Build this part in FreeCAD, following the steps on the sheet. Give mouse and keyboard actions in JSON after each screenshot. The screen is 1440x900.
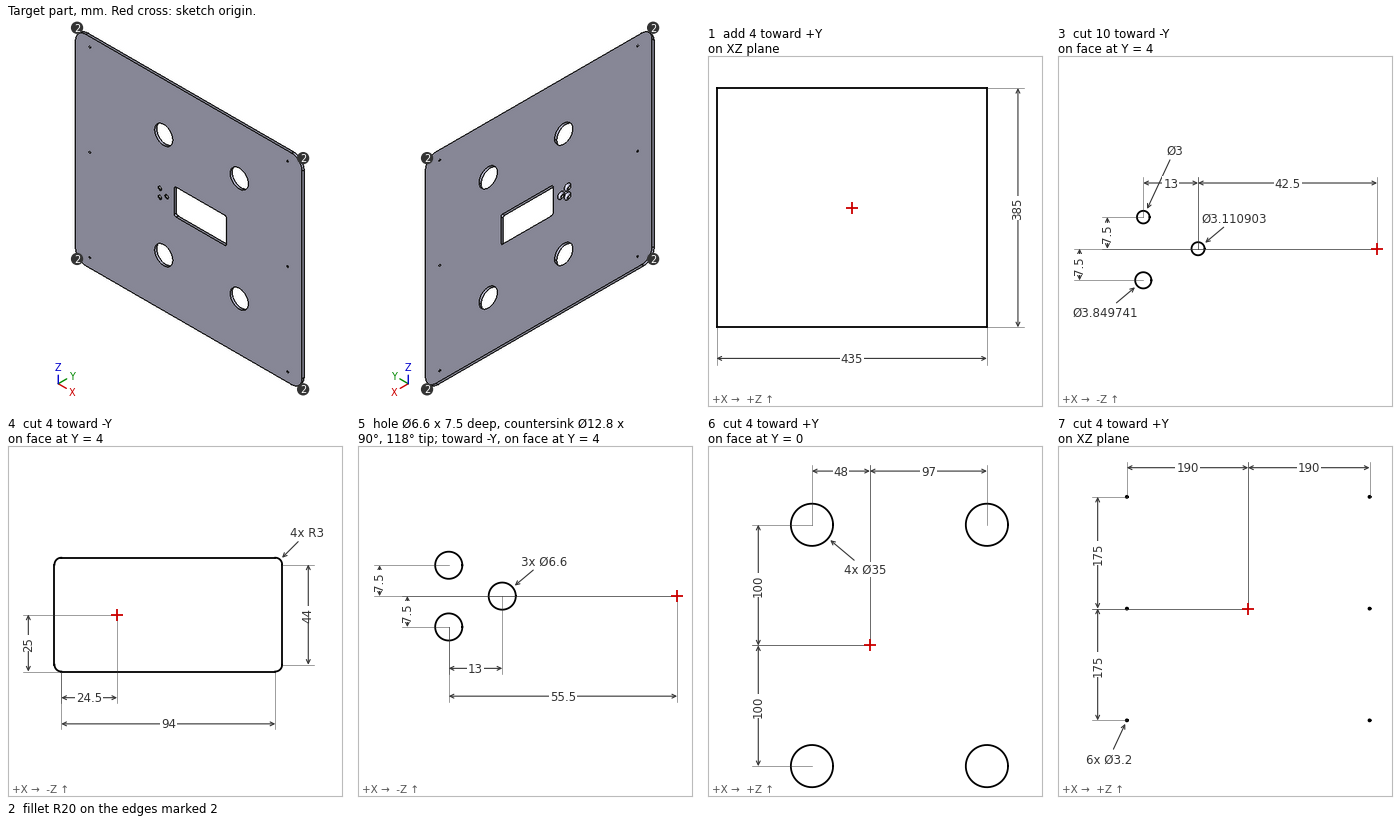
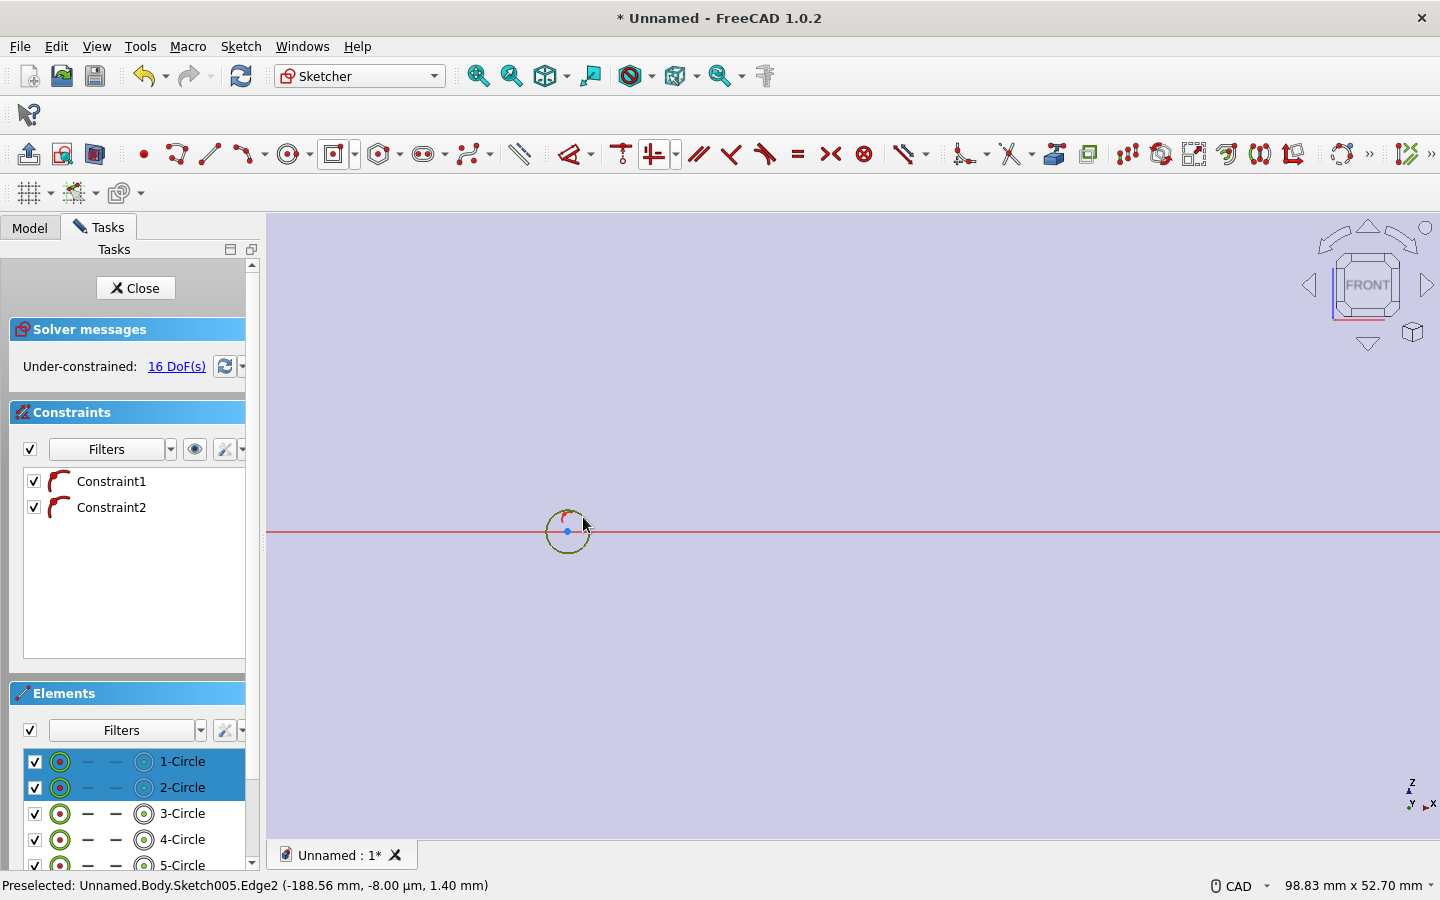
{"action": "scroll", "coordinate": [581, 525], "scroll_direction": "down", "scroll_amount": 12}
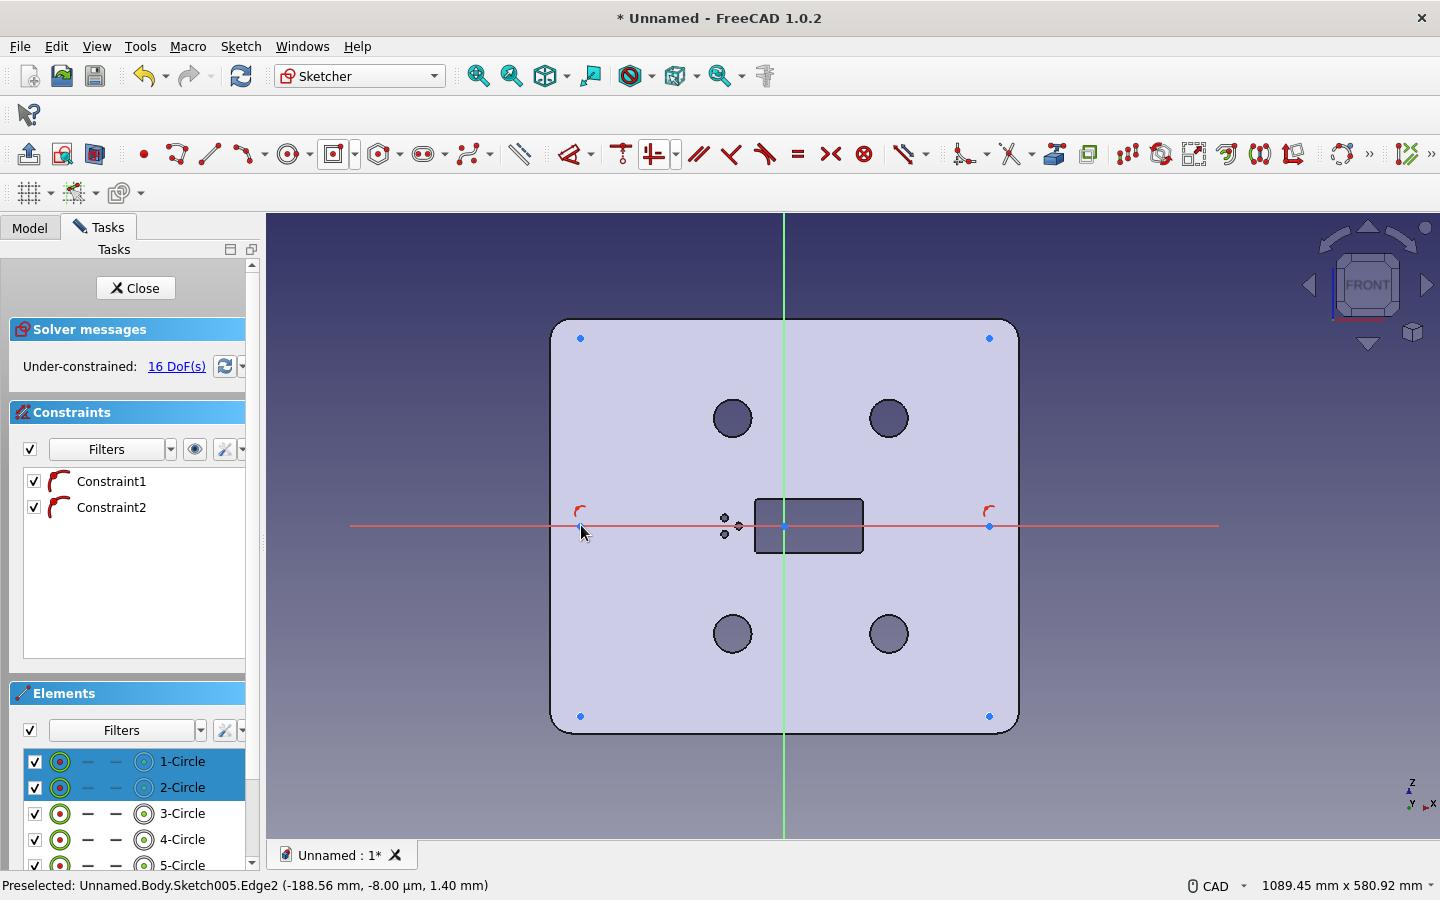
{"action": "scroll", "coordinate": [582, 714], "scroll_direction": "up", "scroll_amount": 9}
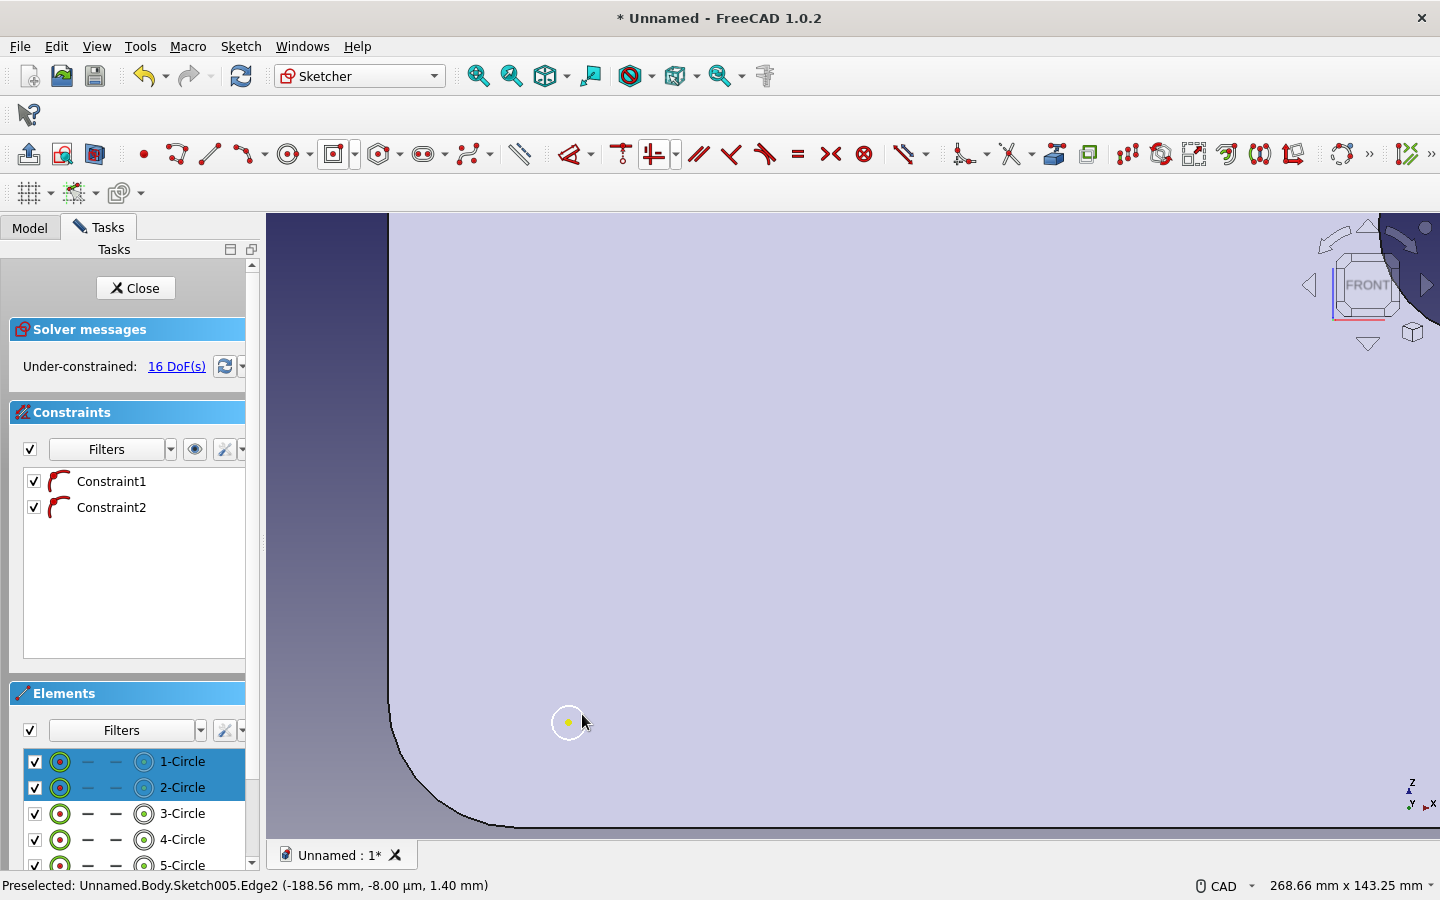
{"action": "left_click", "coordinate": [581, 711]}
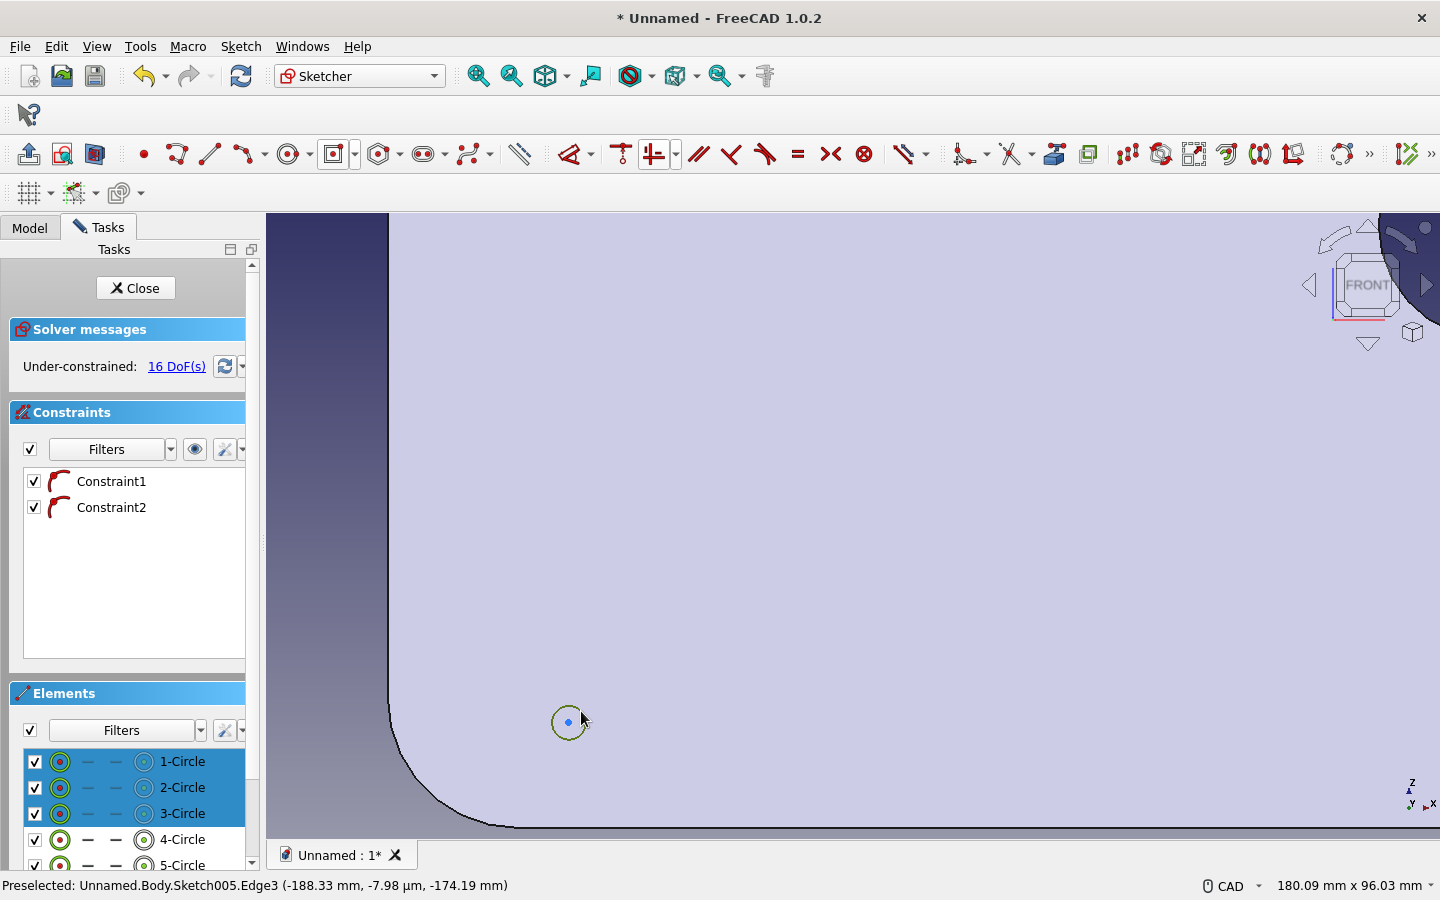
{"action": "scroll", "coordinate": [582, 715], "scroll_direction": "down", "scroll_amount": 9}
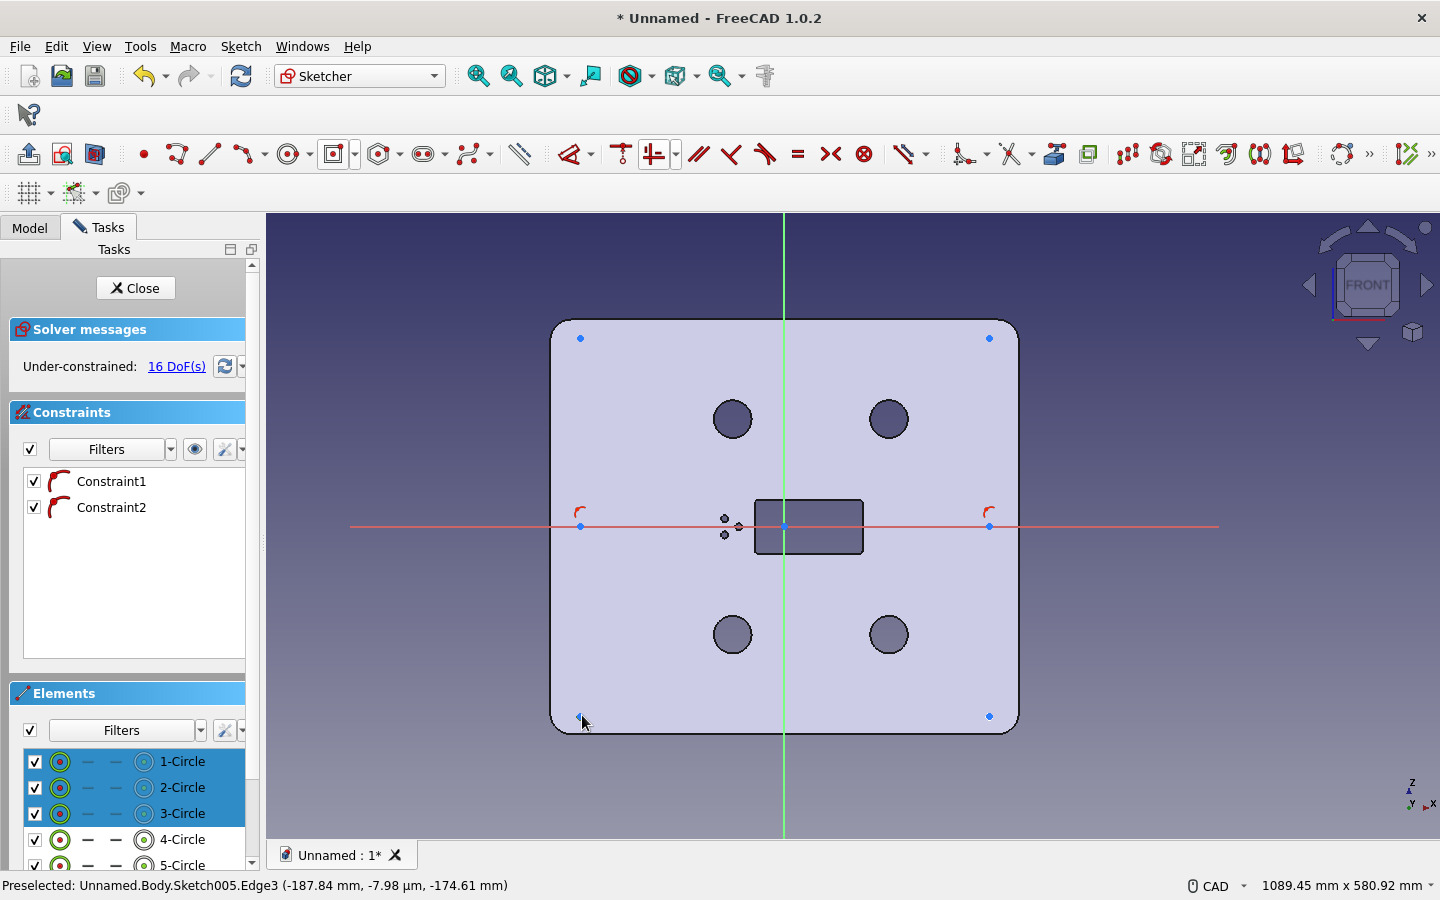
{"action": "scroll", "coordinate": [991, 337], "scroll_direction": "up", "scroll_amount": 10}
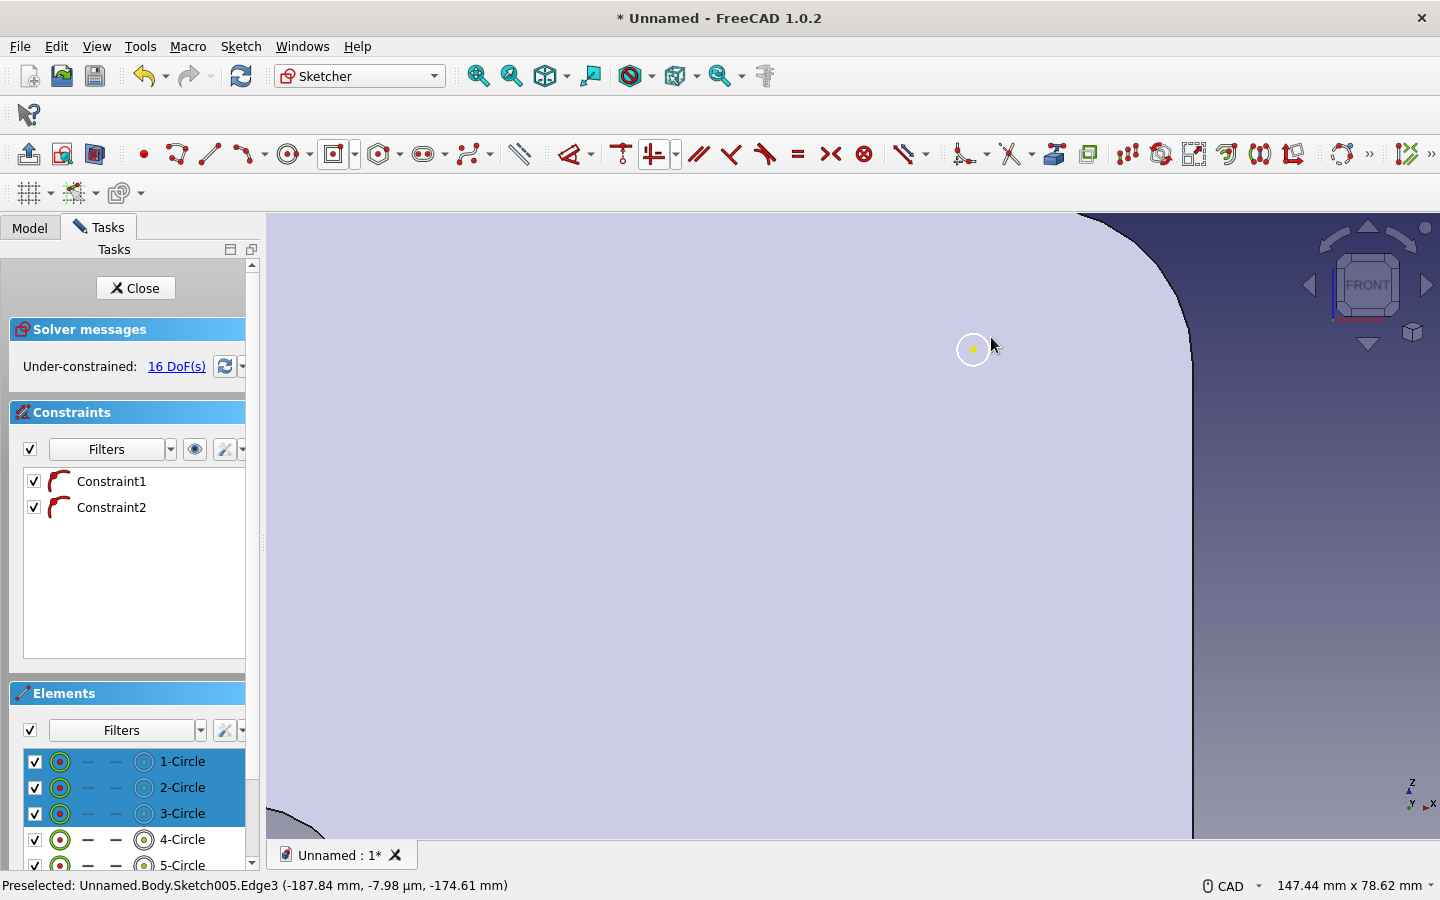
{"action": "left_click", "coordinate": [985, 338]}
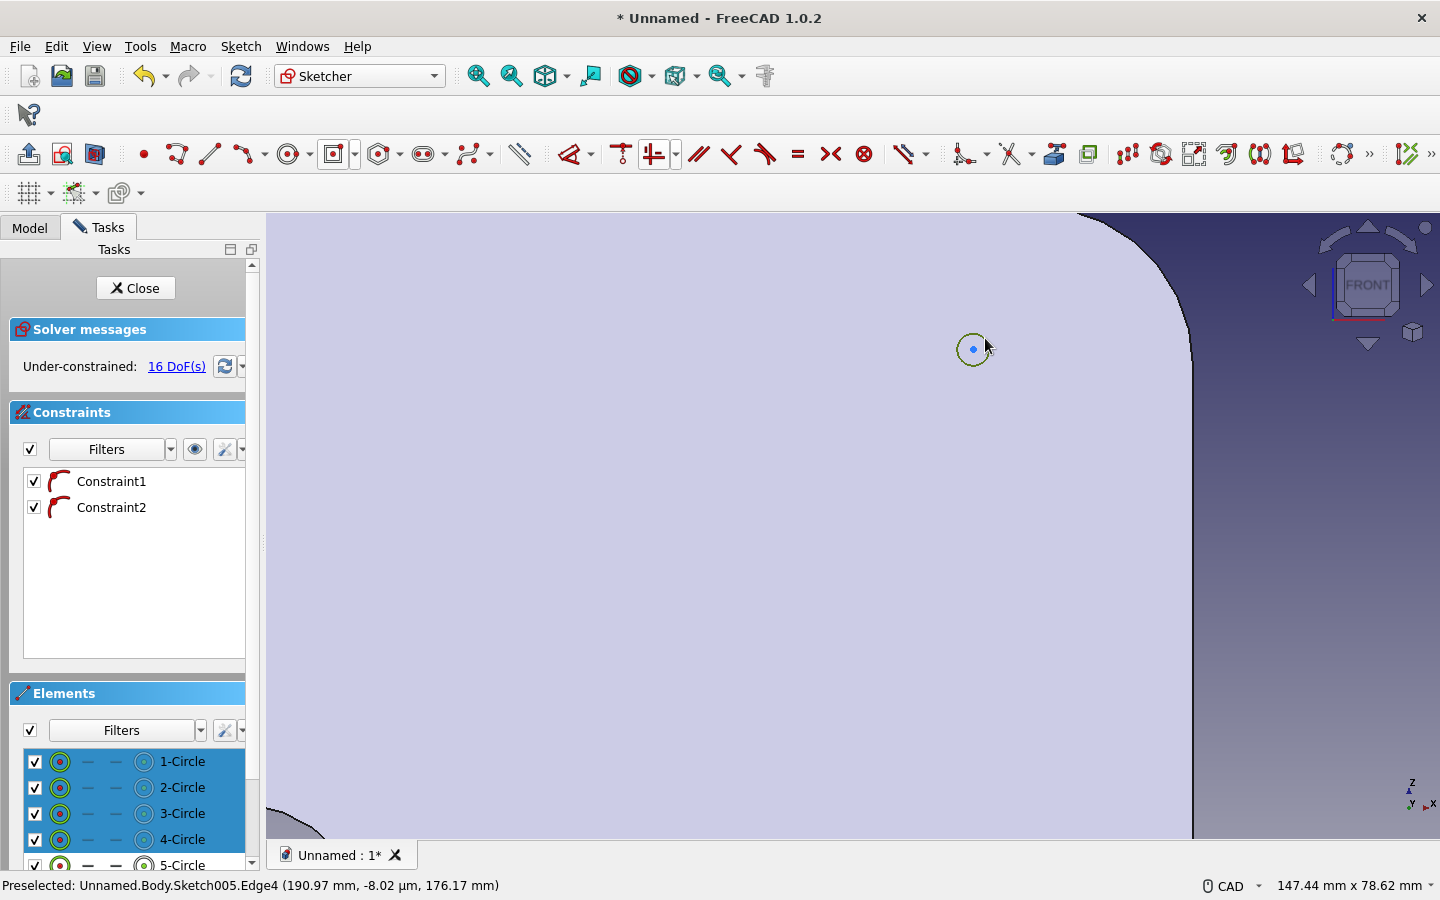
{"action": "scroll", "coordinate": [992, 336], "scroll_direction": "down", "scroll_amount": 10}